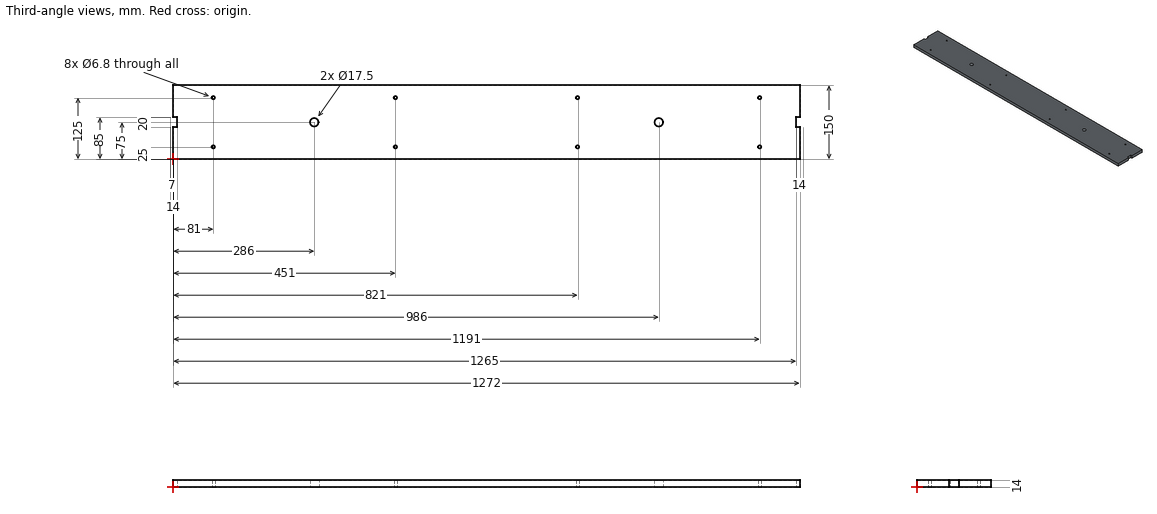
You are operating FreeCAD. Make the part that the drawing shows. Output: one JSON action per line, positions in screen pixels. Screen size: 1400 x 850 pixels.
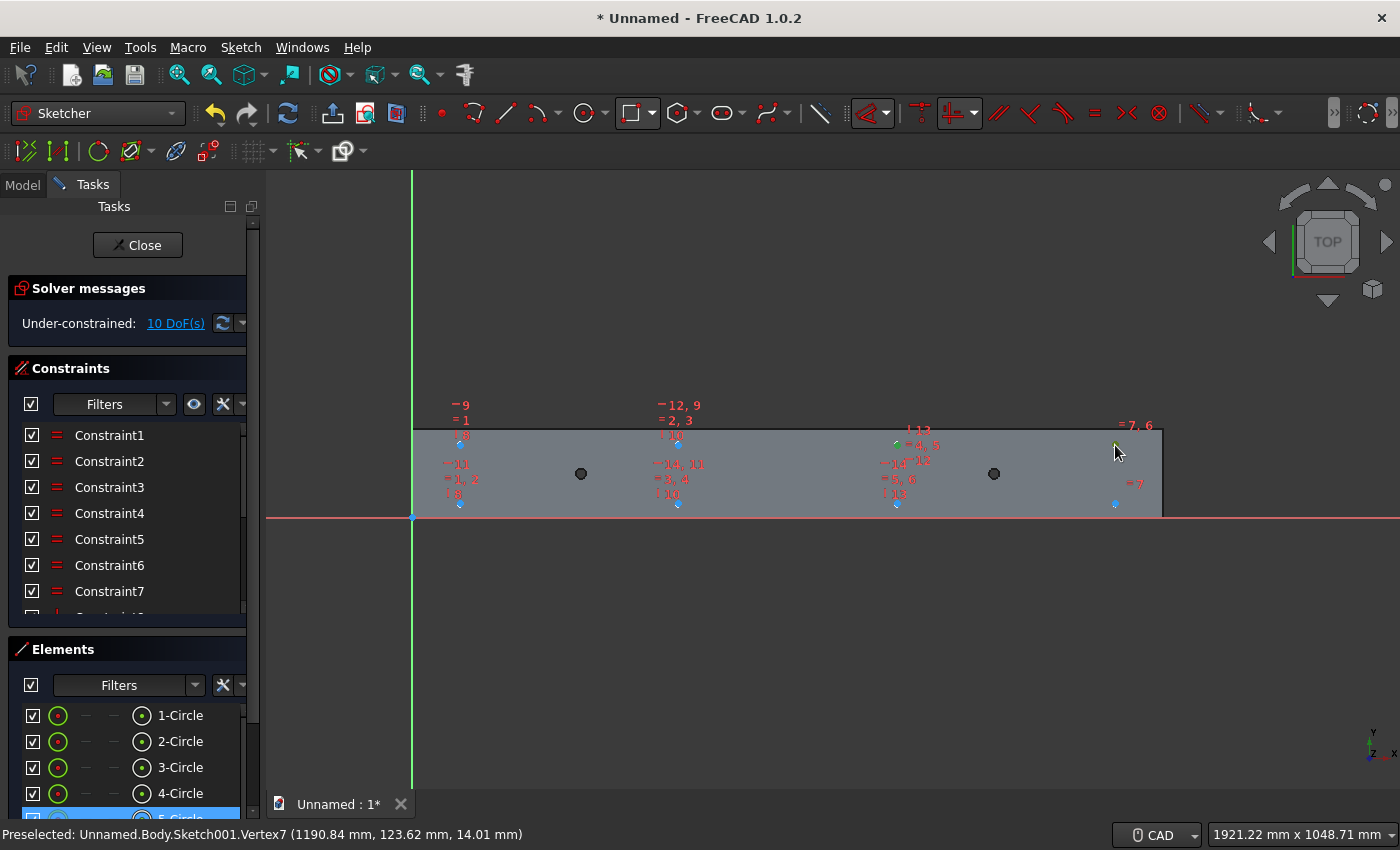
{"action": "left_click", "coordinate": [976, 114]}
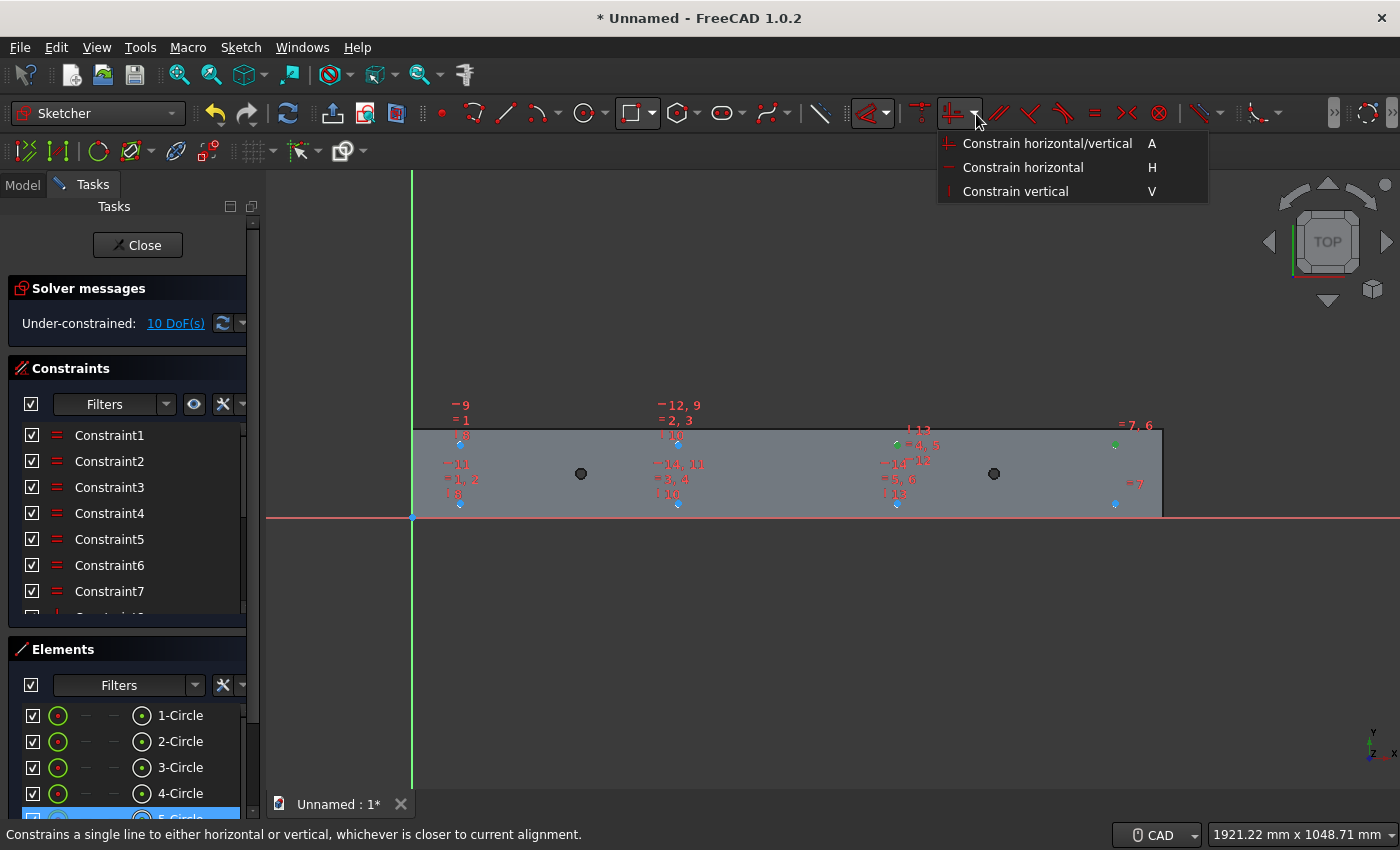
{"action": "left_click", "coordinate": [1073, 167]}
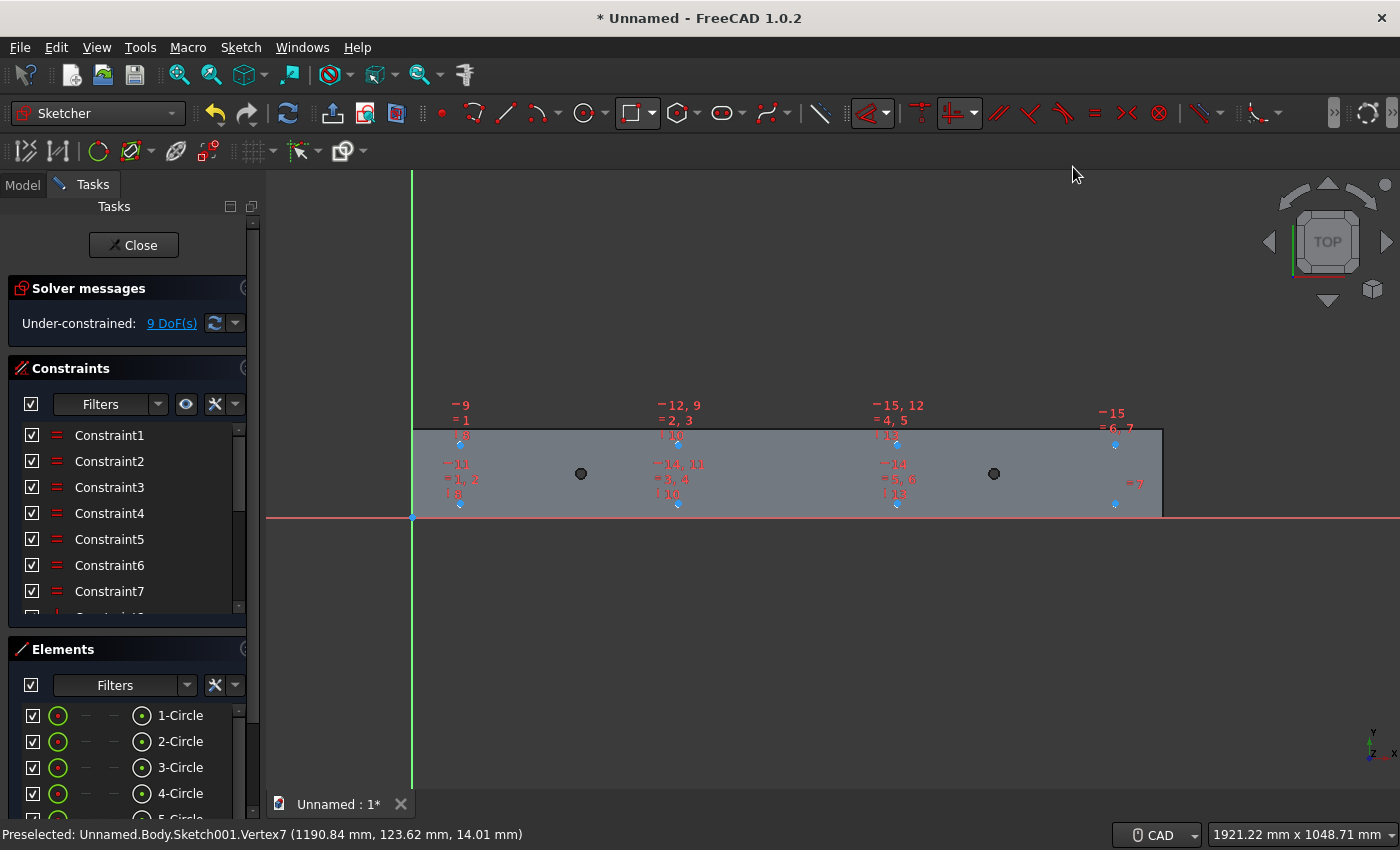
{"action": "left_click", "coordinate": [1115, 445]}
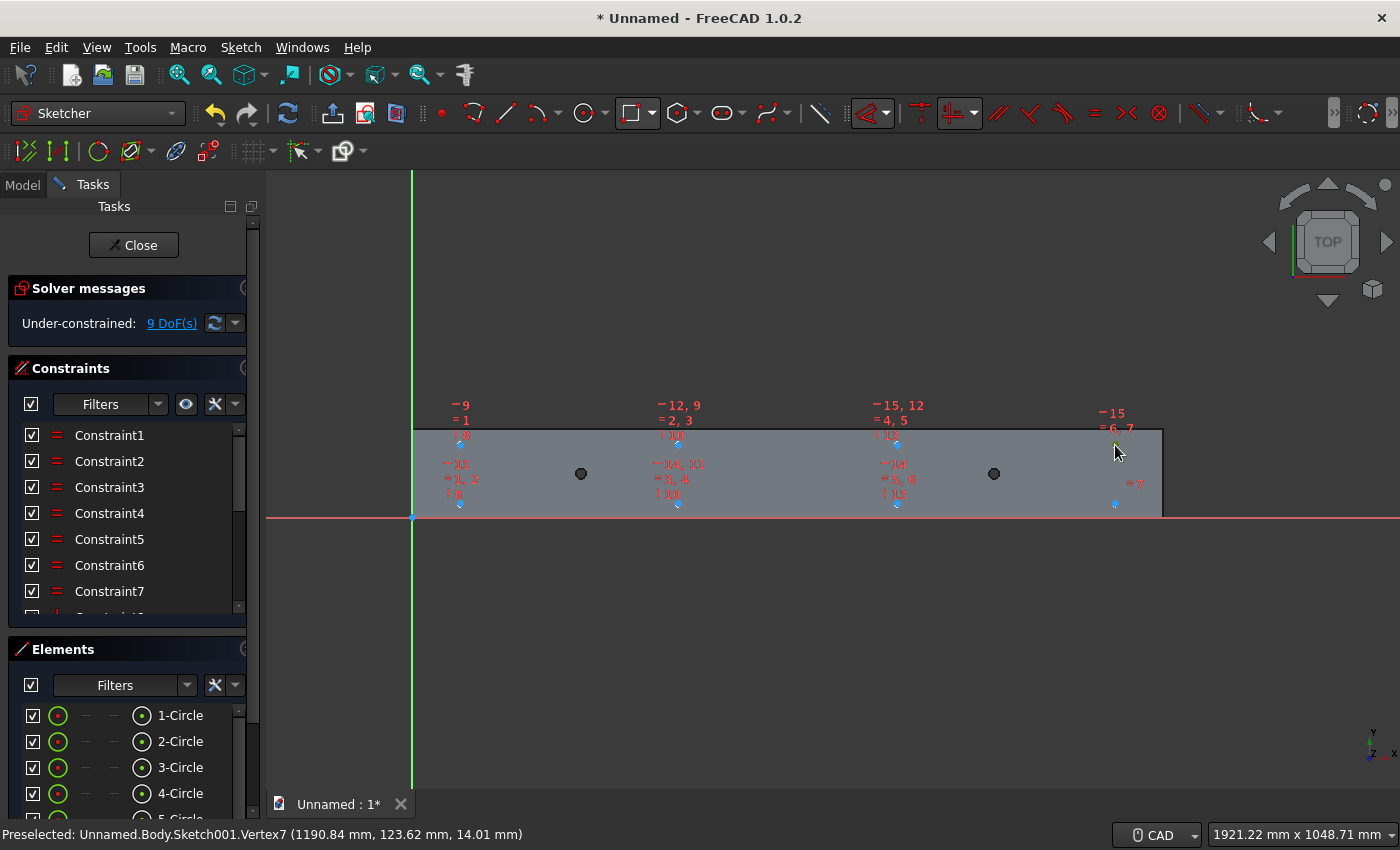
{"action": "left_click", "coordinate": [1115, 504]}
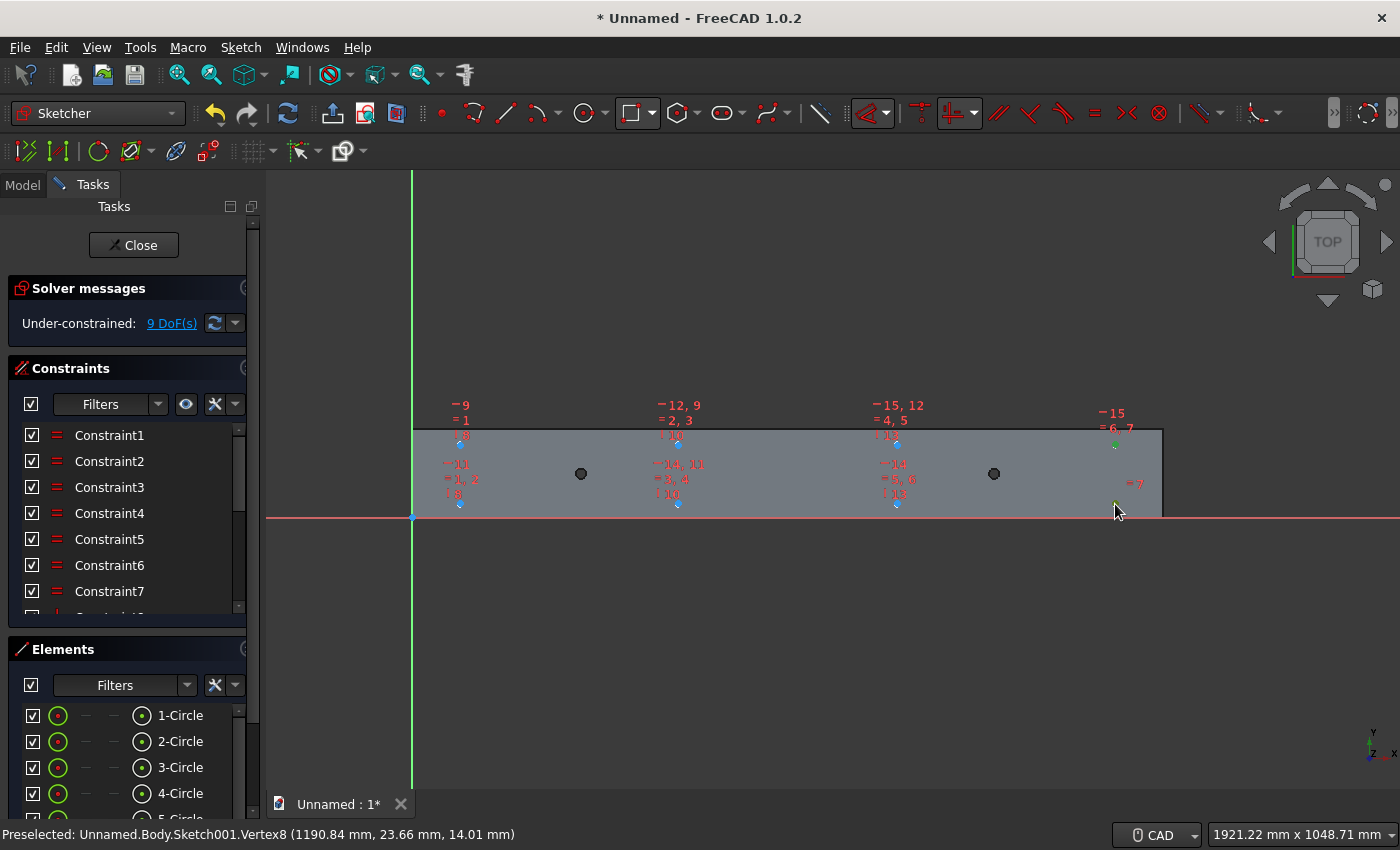
{"action": "left_click", "coordinate": [976, 114]}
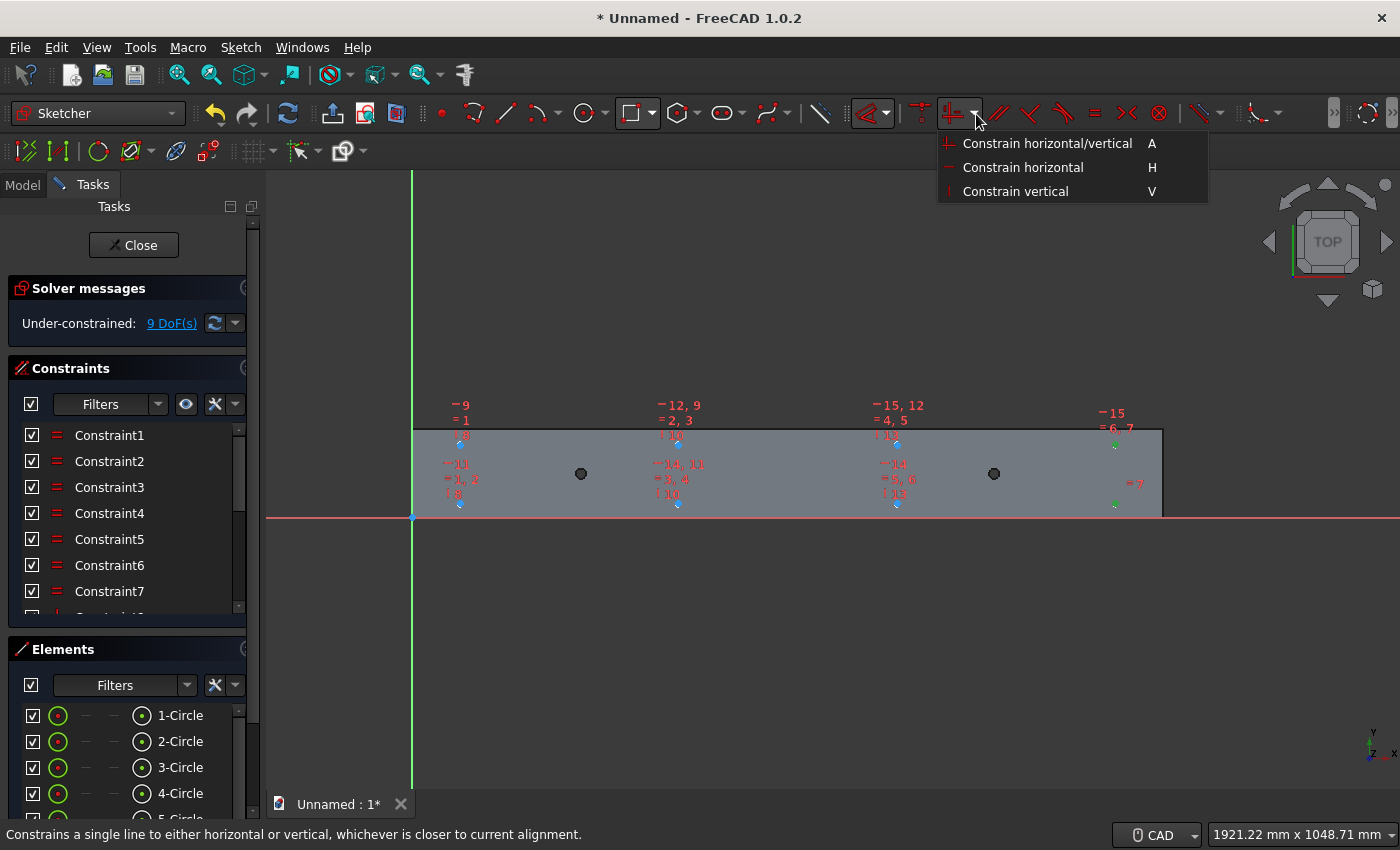
{"action": "left_click", "coordinate": [1073, 191]}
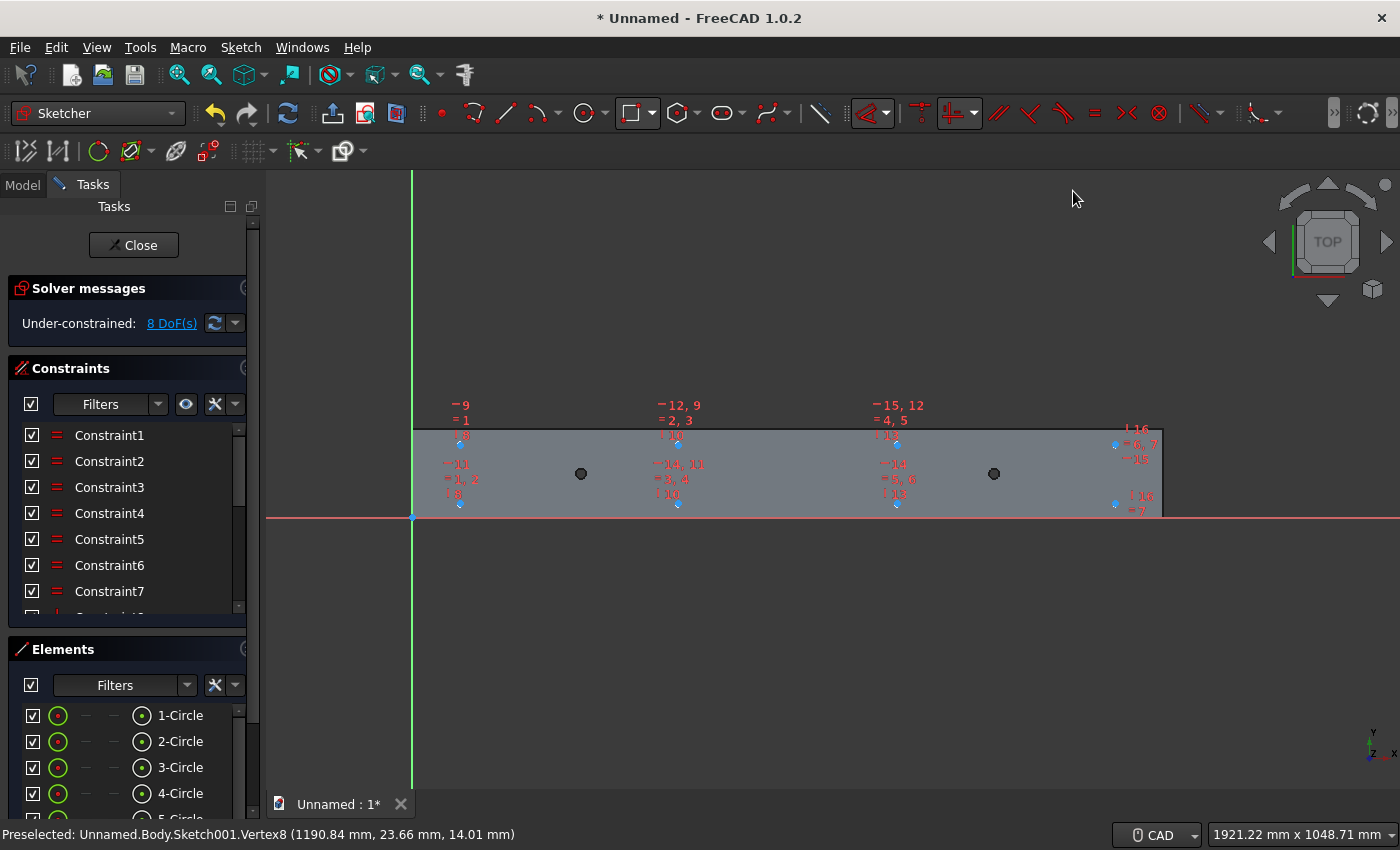
{"action": "left_click", "coordinate": [897, 504]}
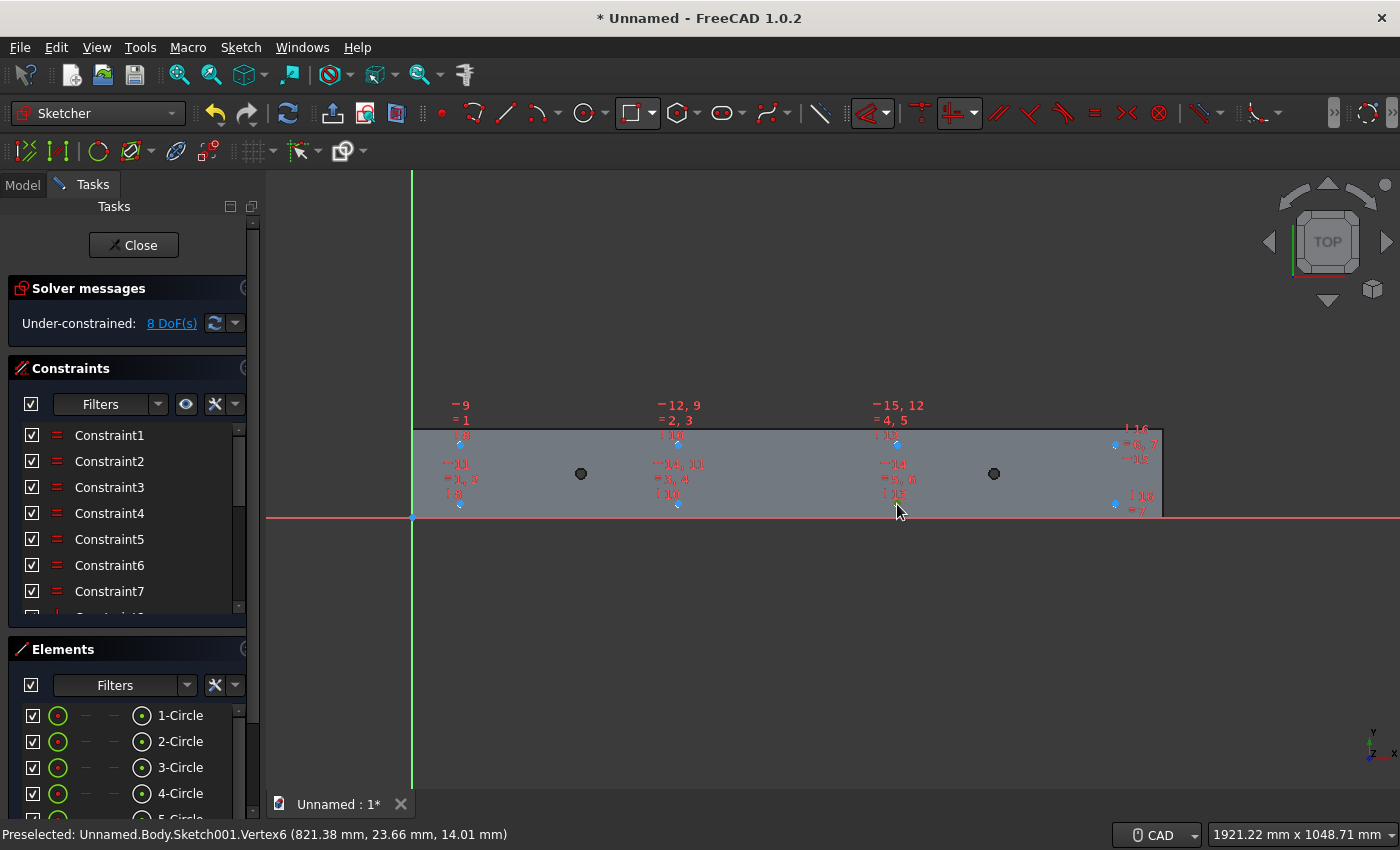
{"action": "left_click", "coordinate": [1115, 504]}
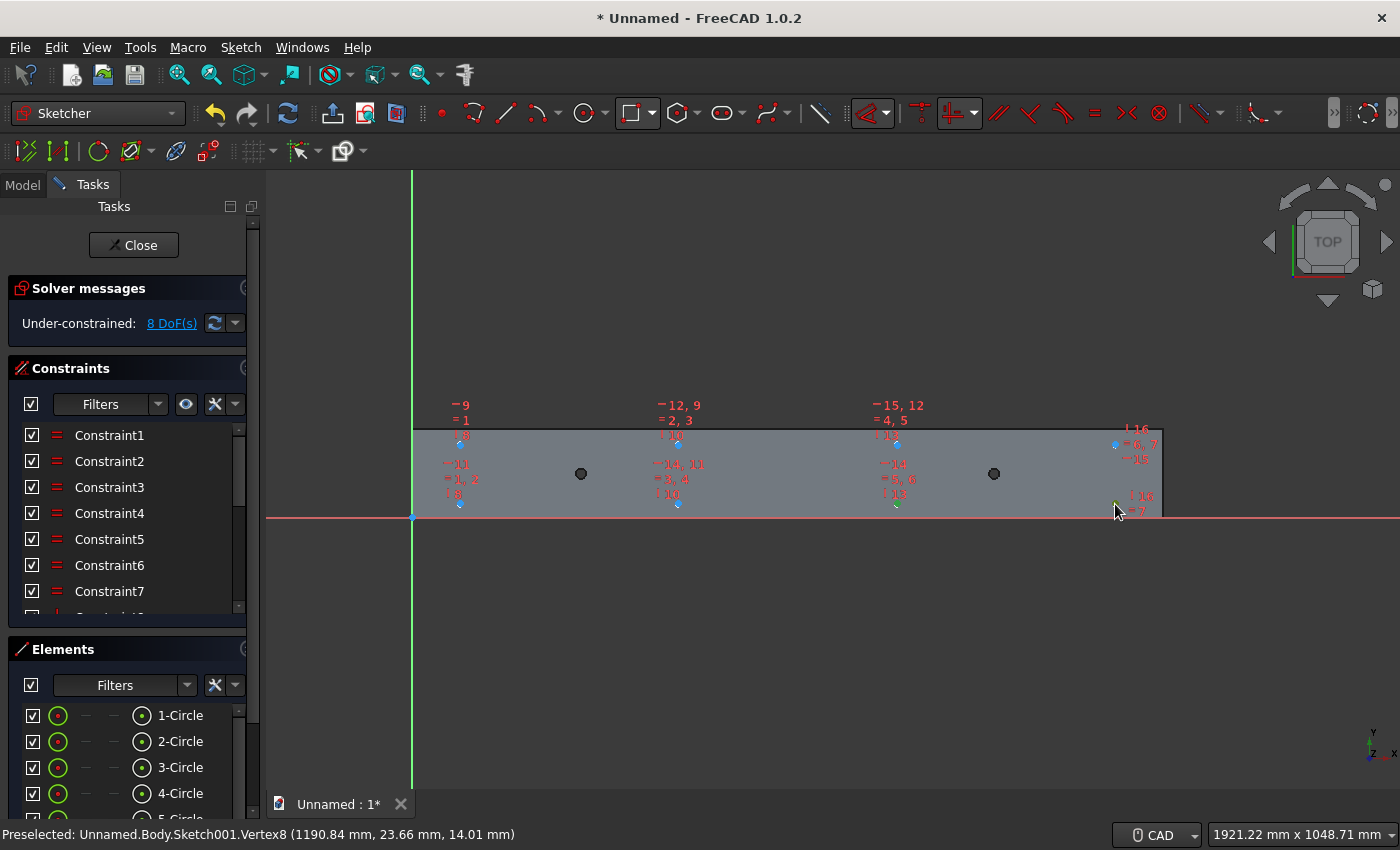
{"action": "key", "text": "h"}